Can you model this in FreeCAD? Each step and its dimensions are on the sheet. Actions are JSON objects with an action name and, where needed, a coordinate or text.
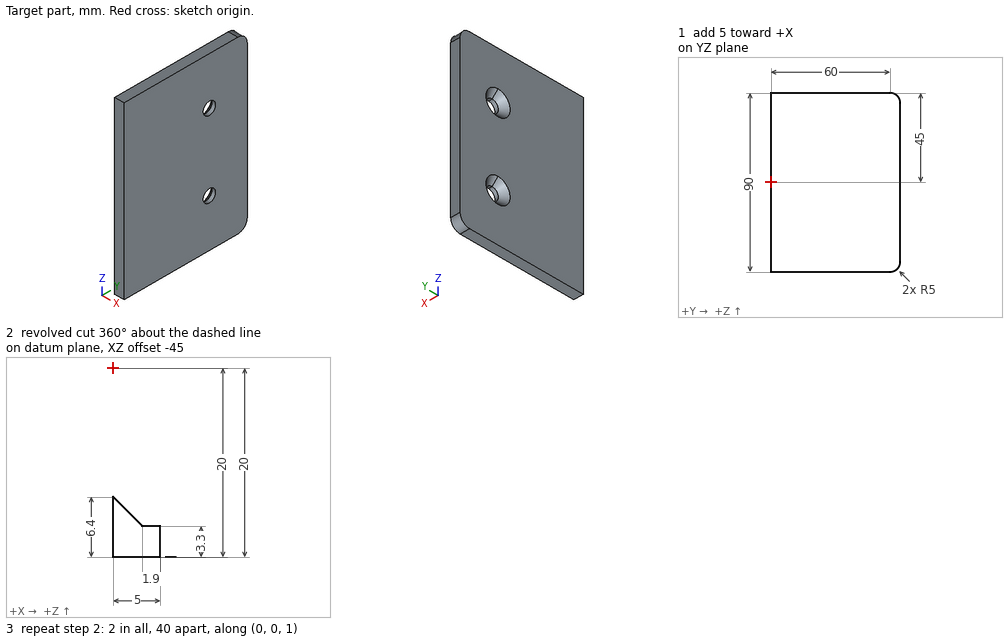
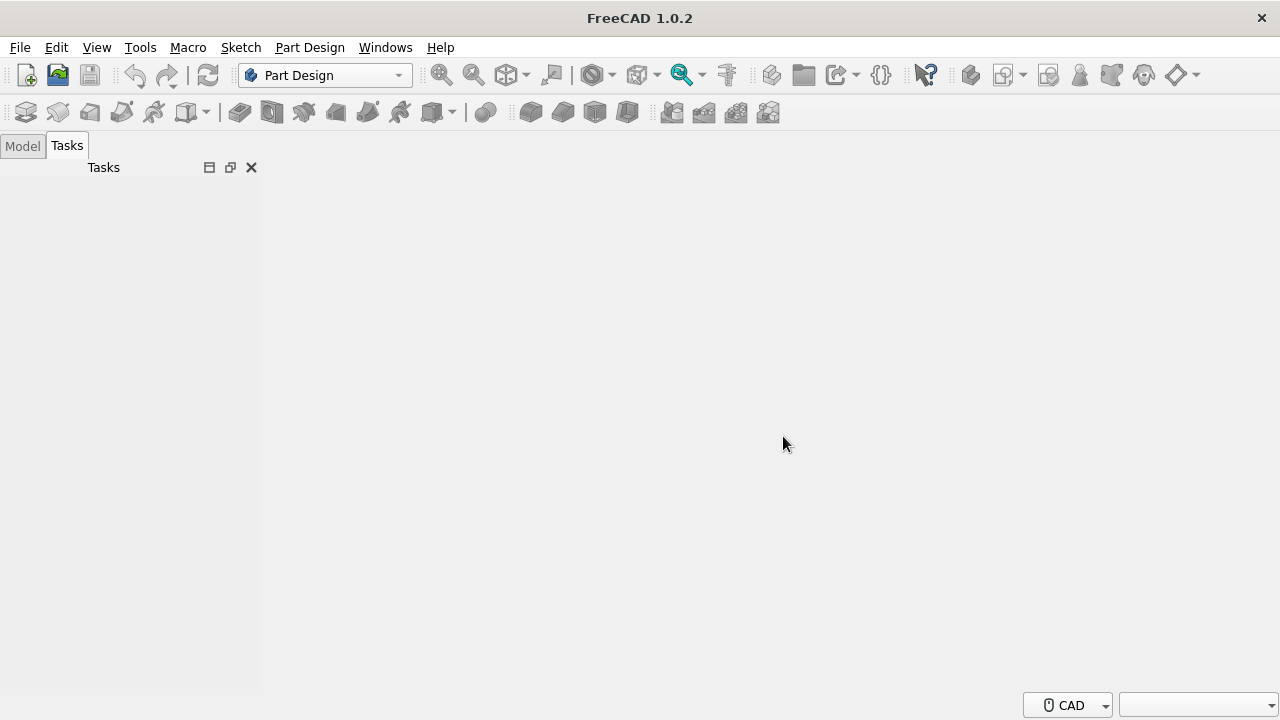
{"action": "key", "text": "ctrl+n"}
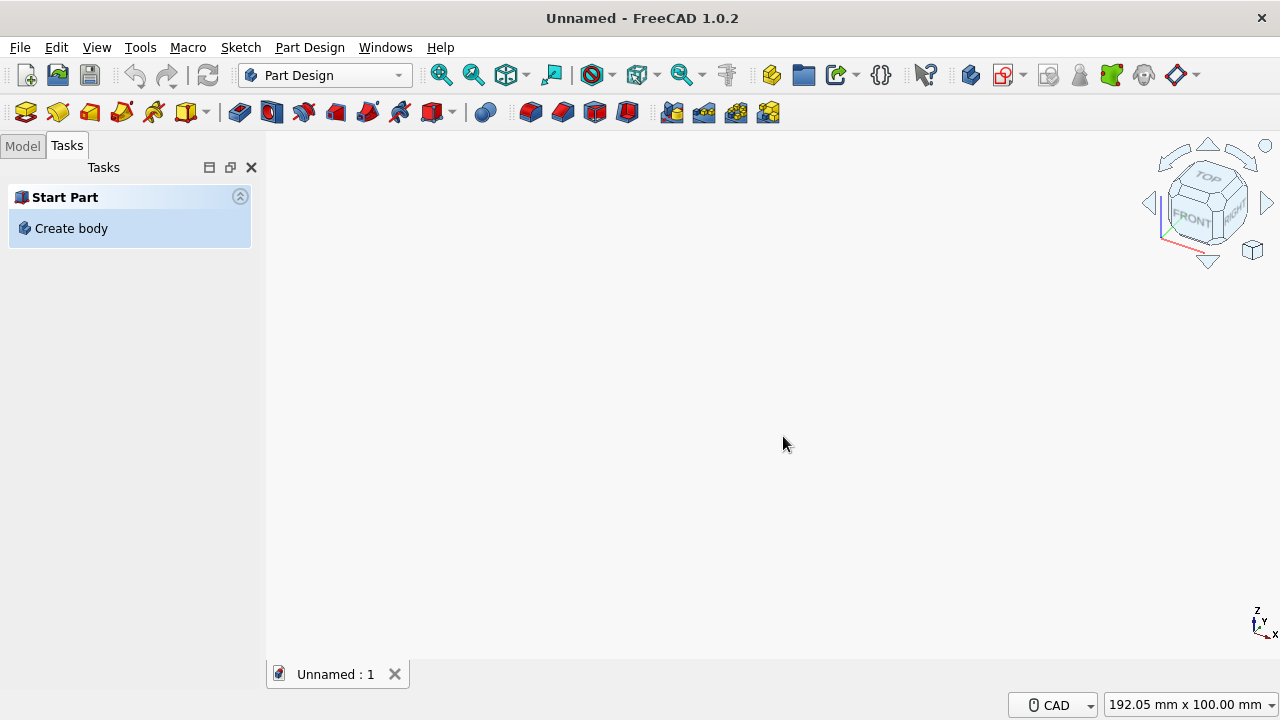
{"action": "left_click", "coordinate": [1004, 76]}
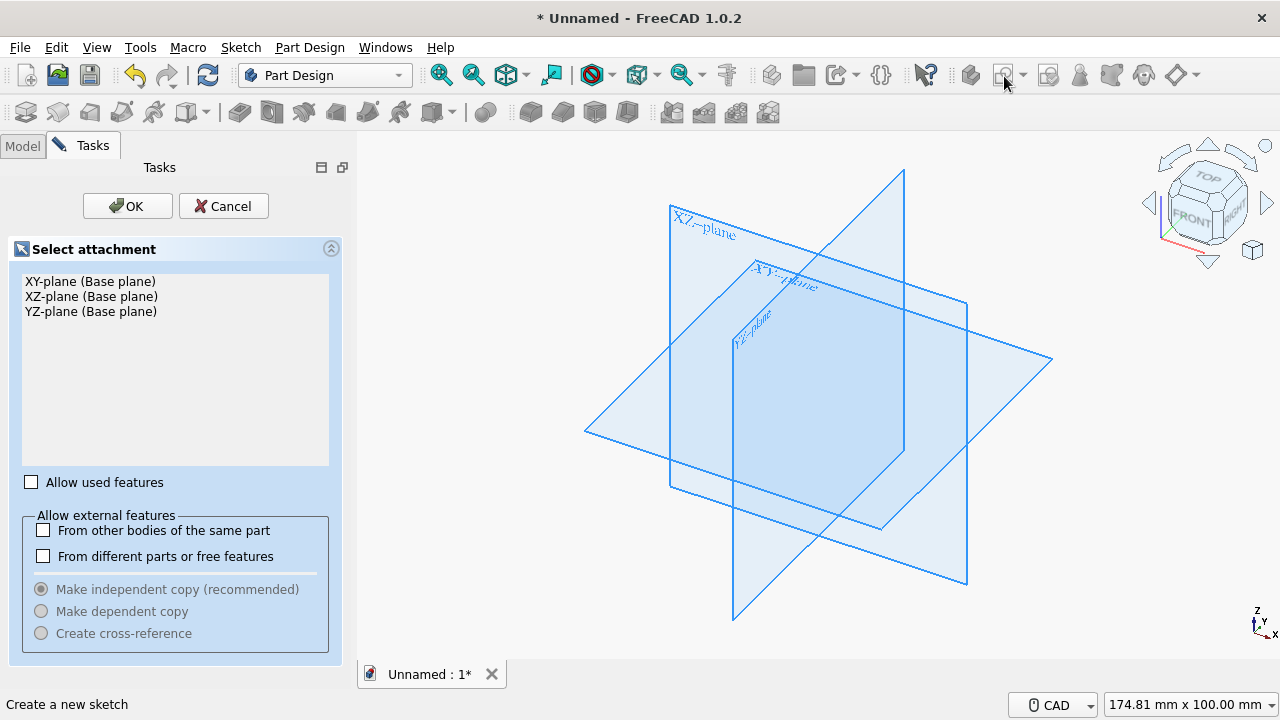
{"action": "left_click", "coordinate": [82, 312]}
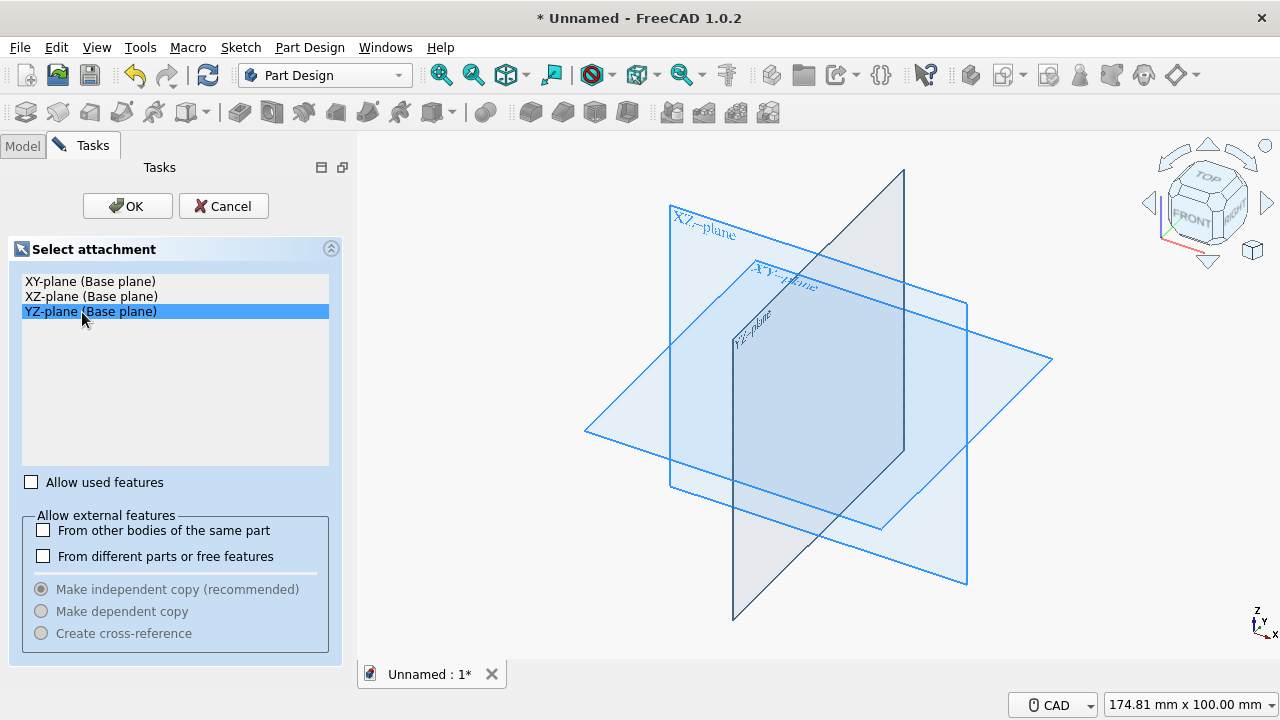
{"action": "left_click", "coordinate": [128, 206]}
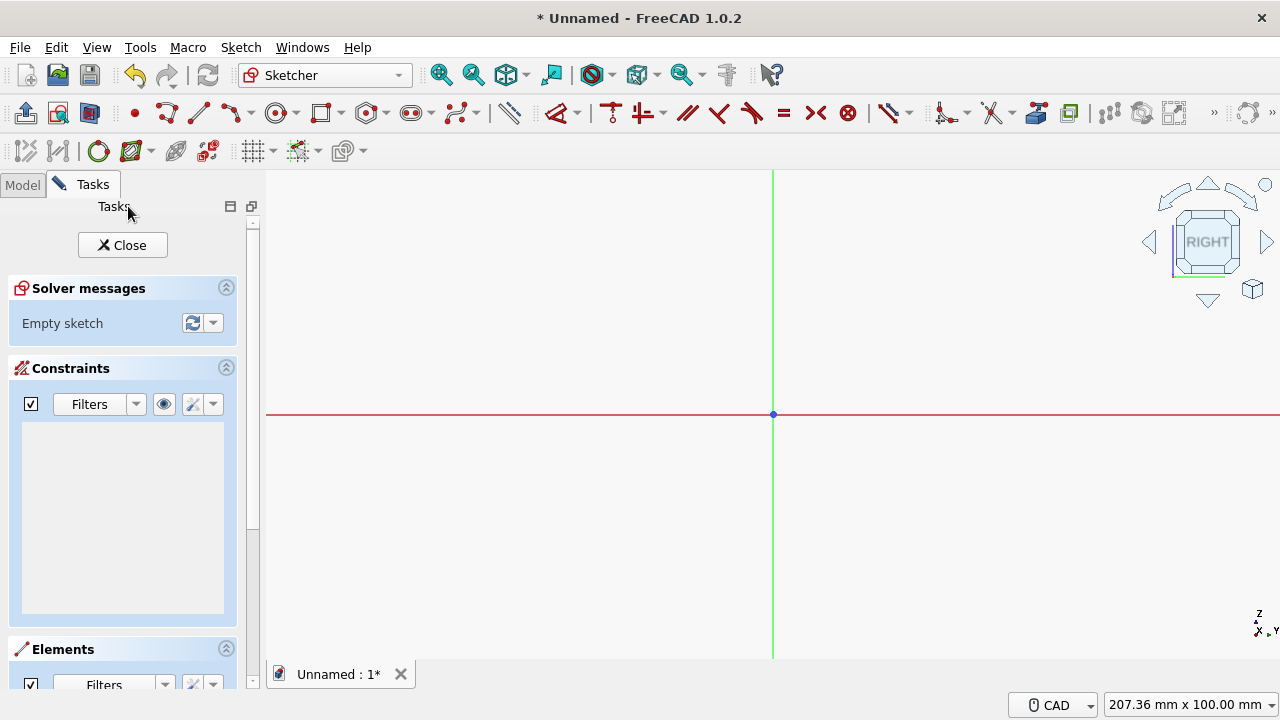
{"action": "scroll", "coordinate": [294, 414], "scroll_direction": "down", "scroll_amount": 2}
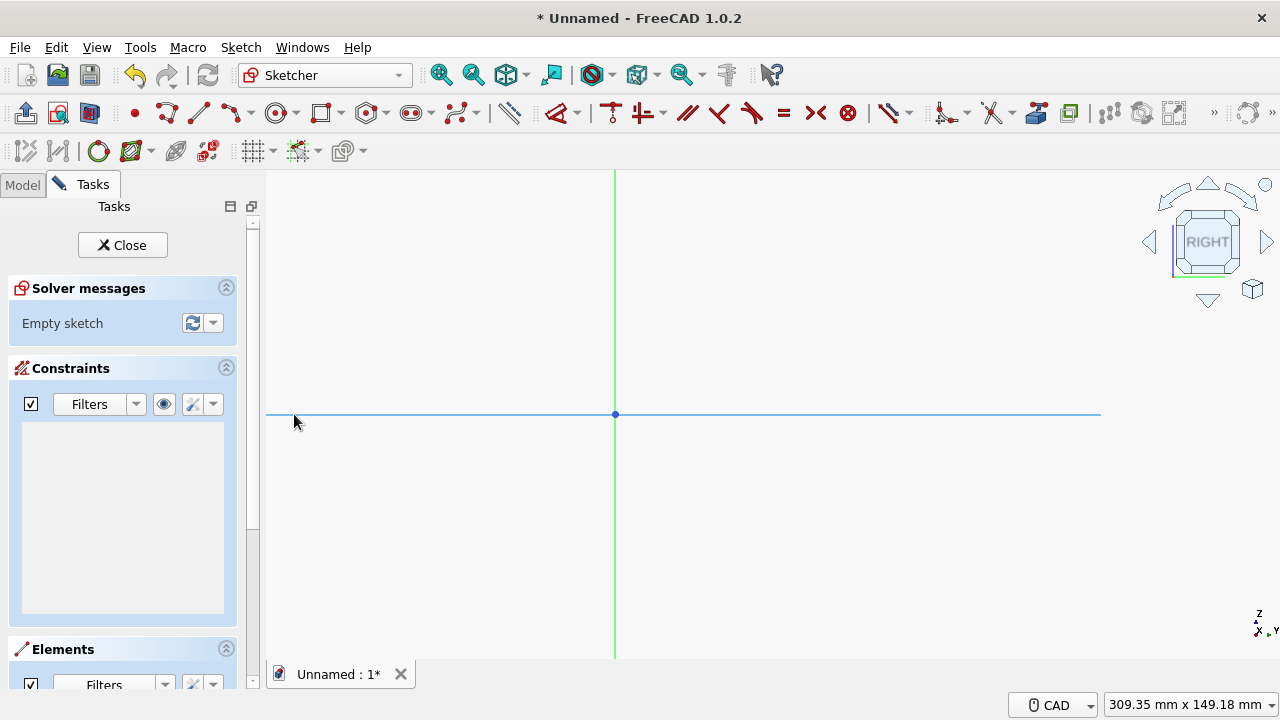
{"action": "left_click", "coordinate": [168, 114]}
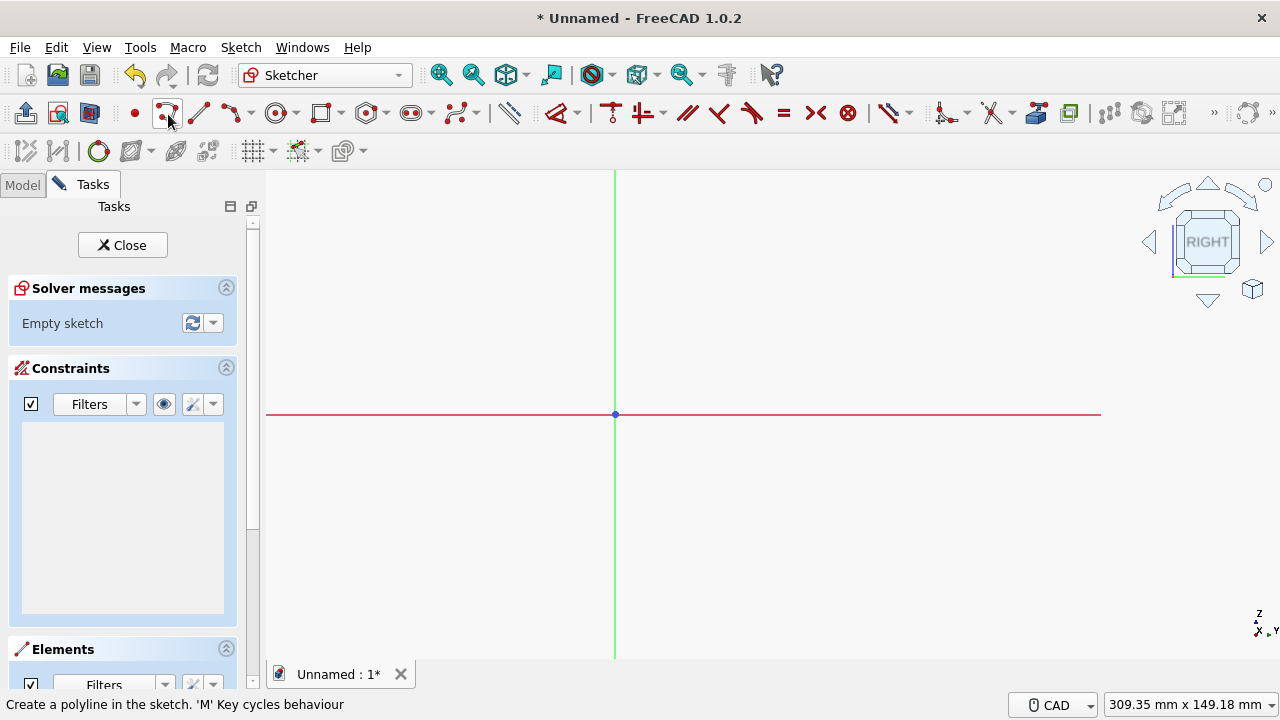
{"action": "left_click", "coordinate": [812, 267]}
{"action": "left_click", "coordinate": [615, 267]}
{"action": "left_click", "coordinate": [624, 562]}
{"action": "left_click", "coordinate": [812, 562]}
{"action": "right_click", "coordinate": [812, 562]}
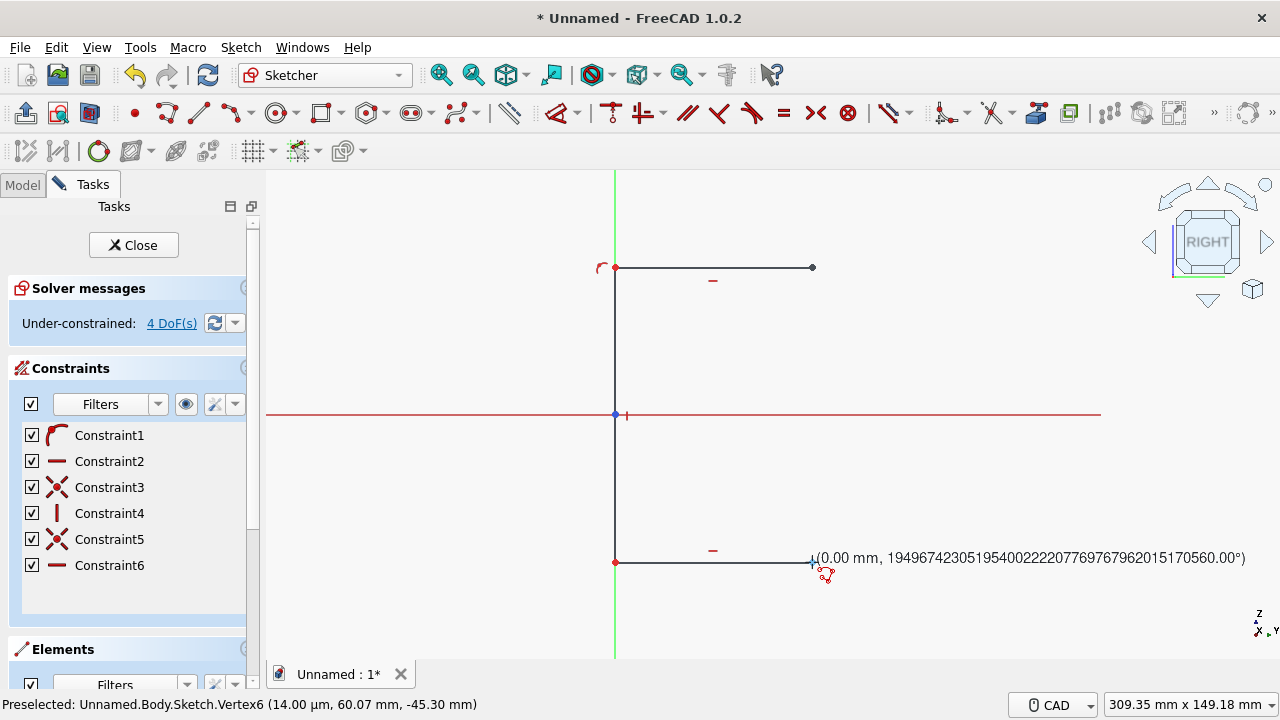
{"action": "left_click", "coordinate": [200, 114]}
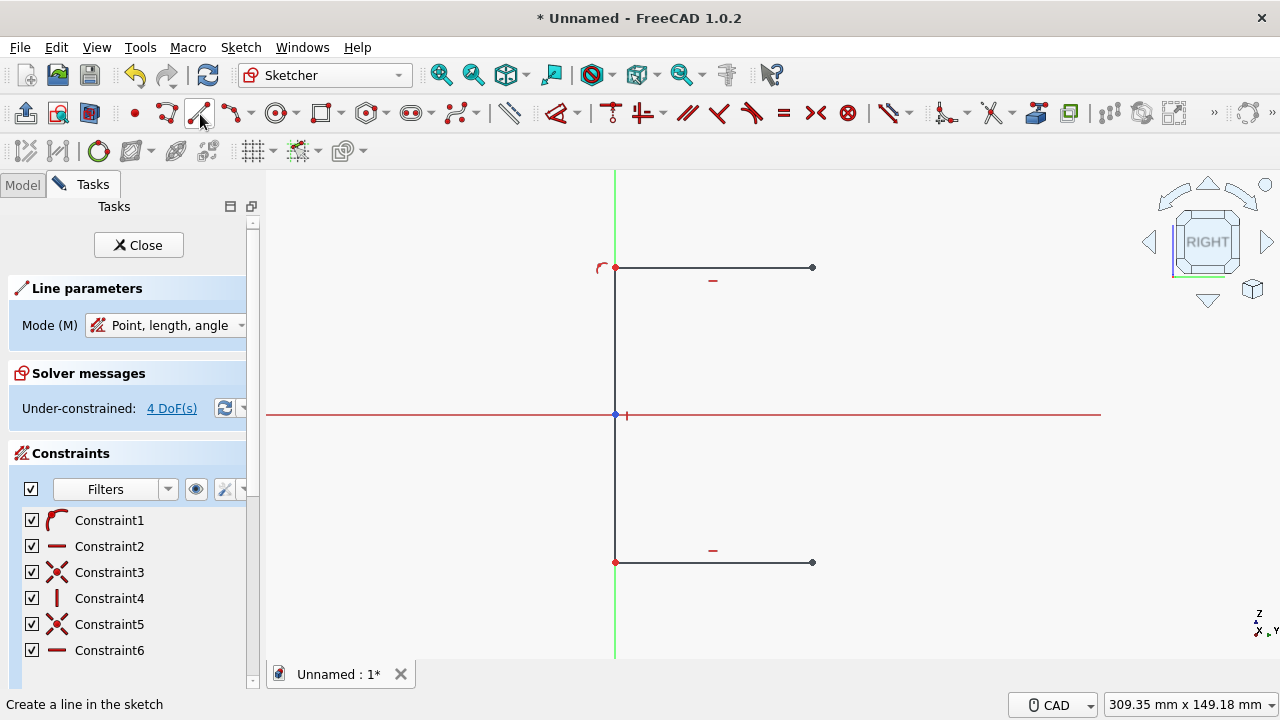
{"action": "left_click", "coordinate": [828, 546]}
{"action": "left_click", "coordinate": [828, 283]}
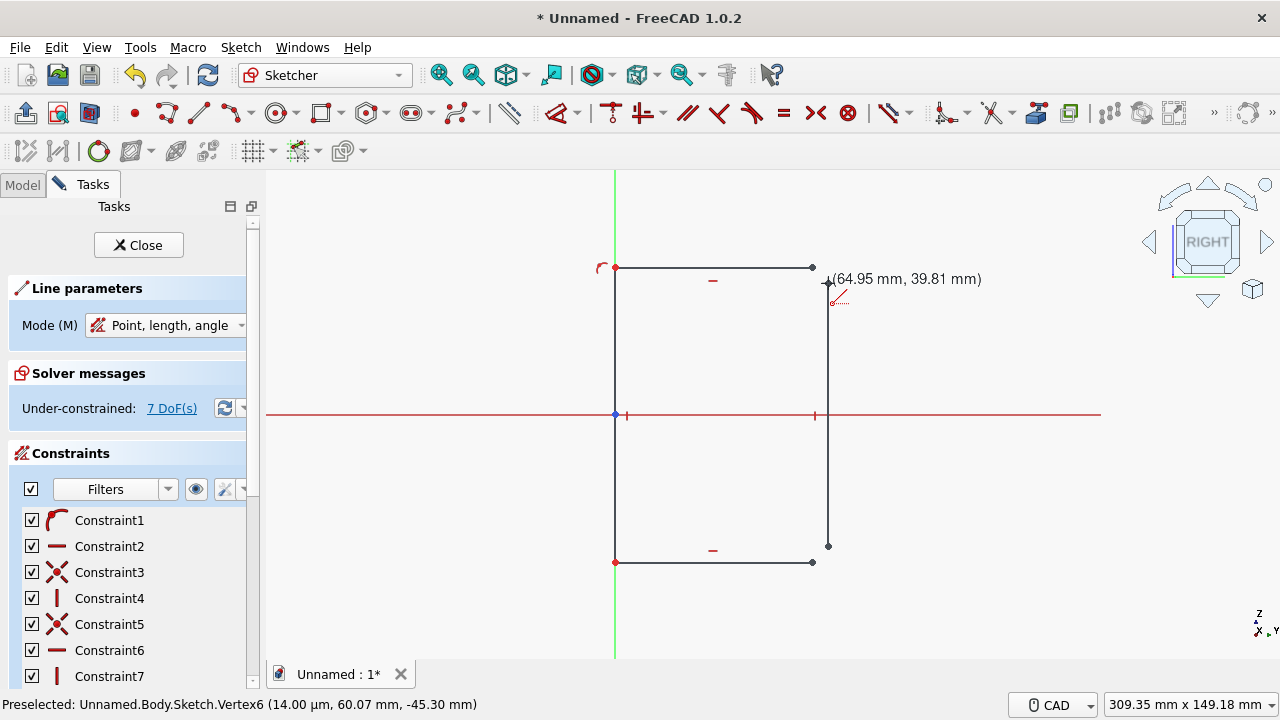
{"action": "key", "text": "g 3 a"}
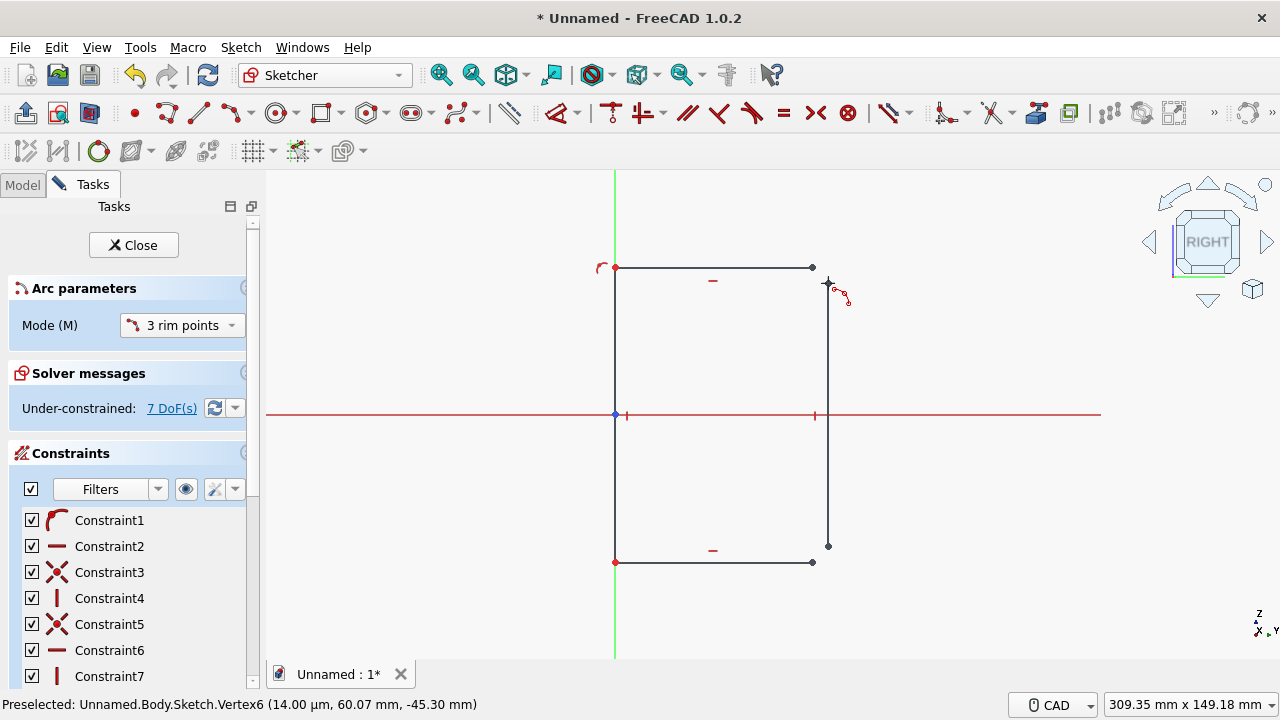
{"action": "left_click", "coordinate": [812, 563]}
{"action": "left_click", "coordinate": [828, 547]}